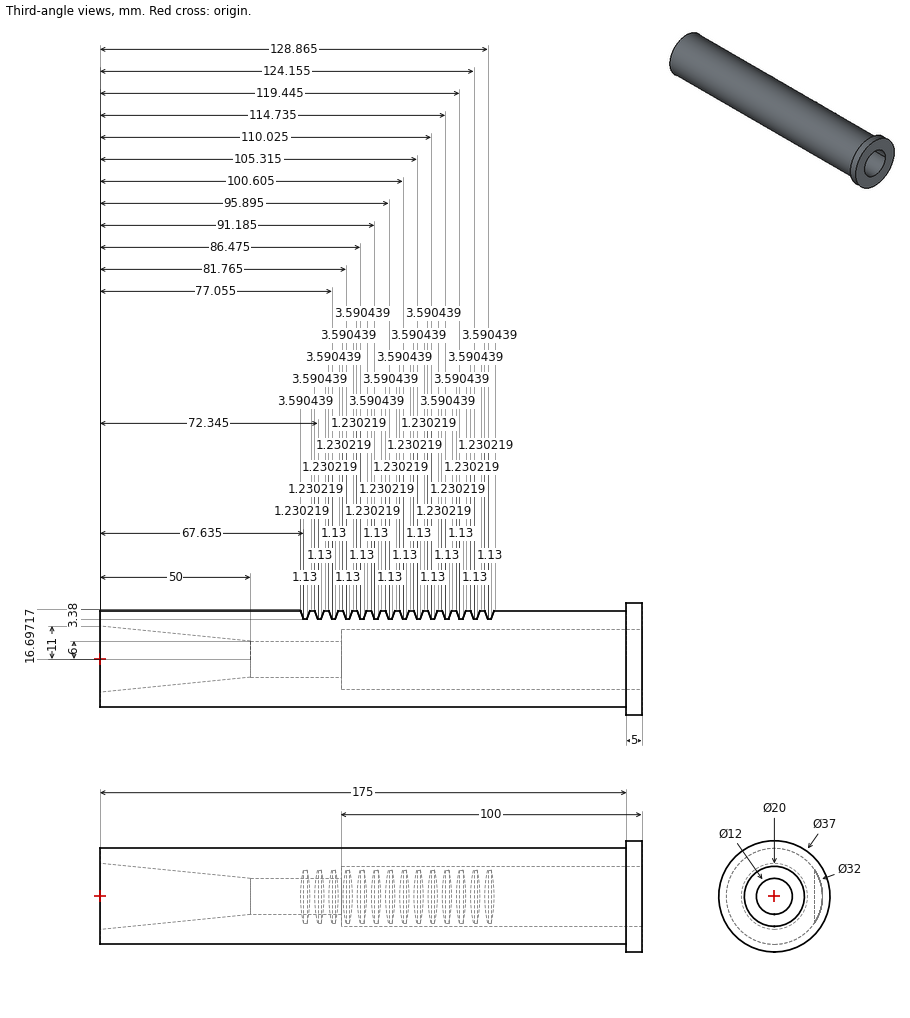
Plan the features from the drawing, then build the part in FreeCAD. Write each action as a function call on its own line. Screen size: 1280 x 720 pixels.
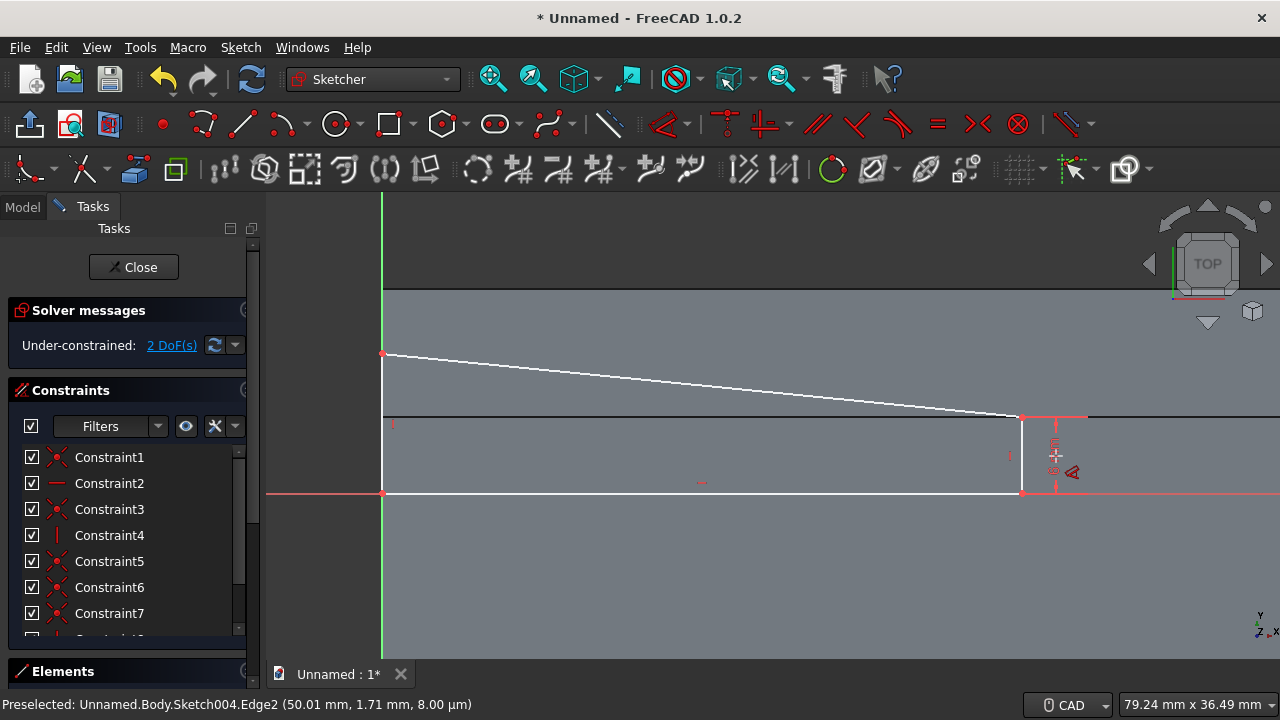
click(574, 494)
click(702, 528)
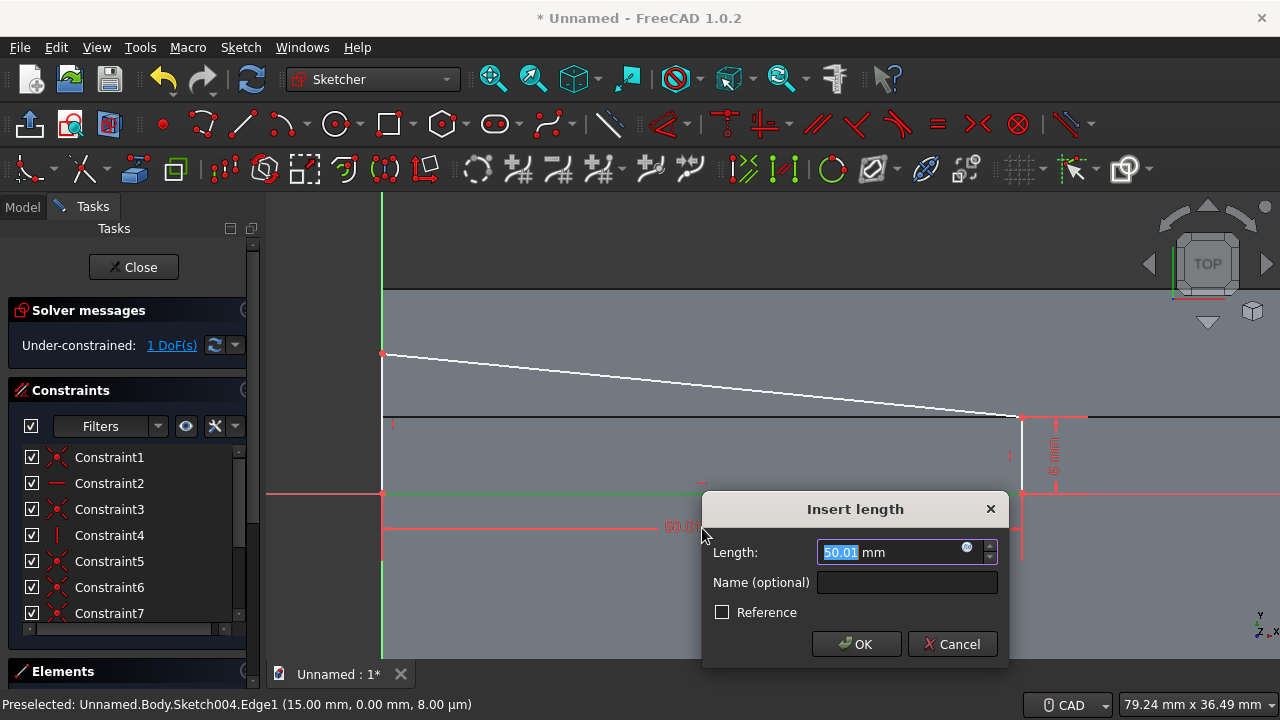
text(50)
key(Return)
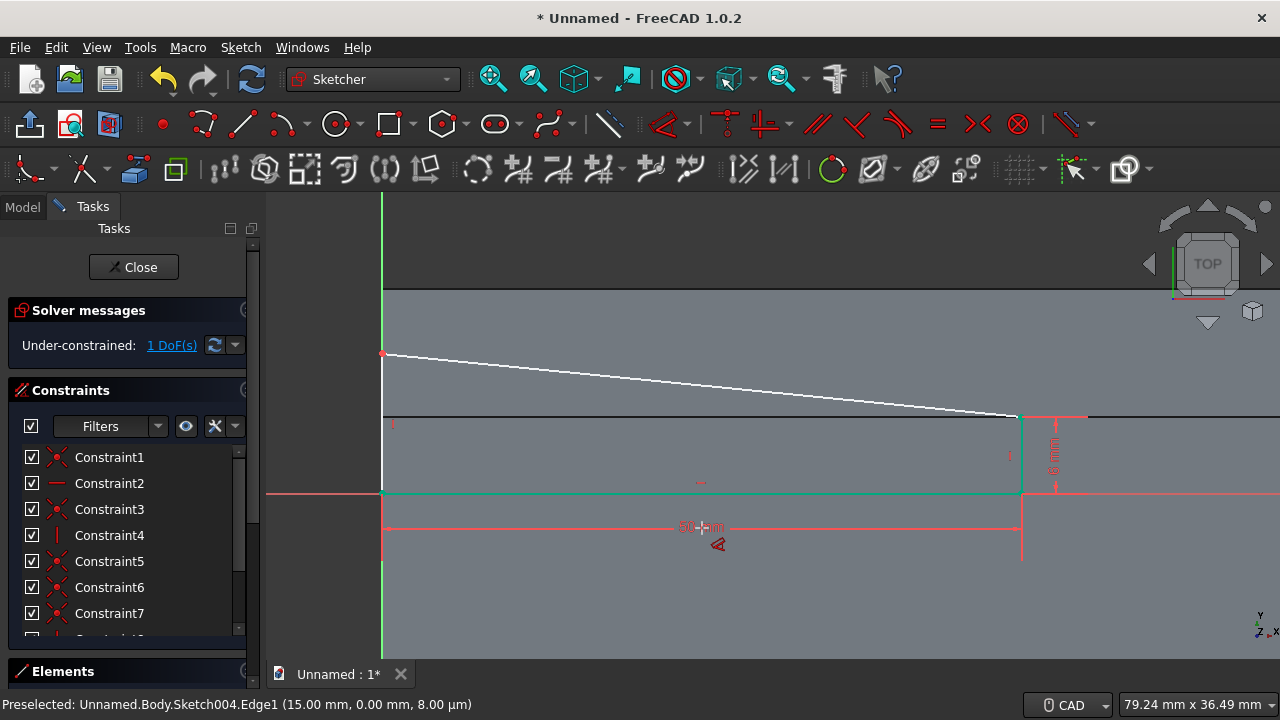
click(382, 396)
click(348, 424)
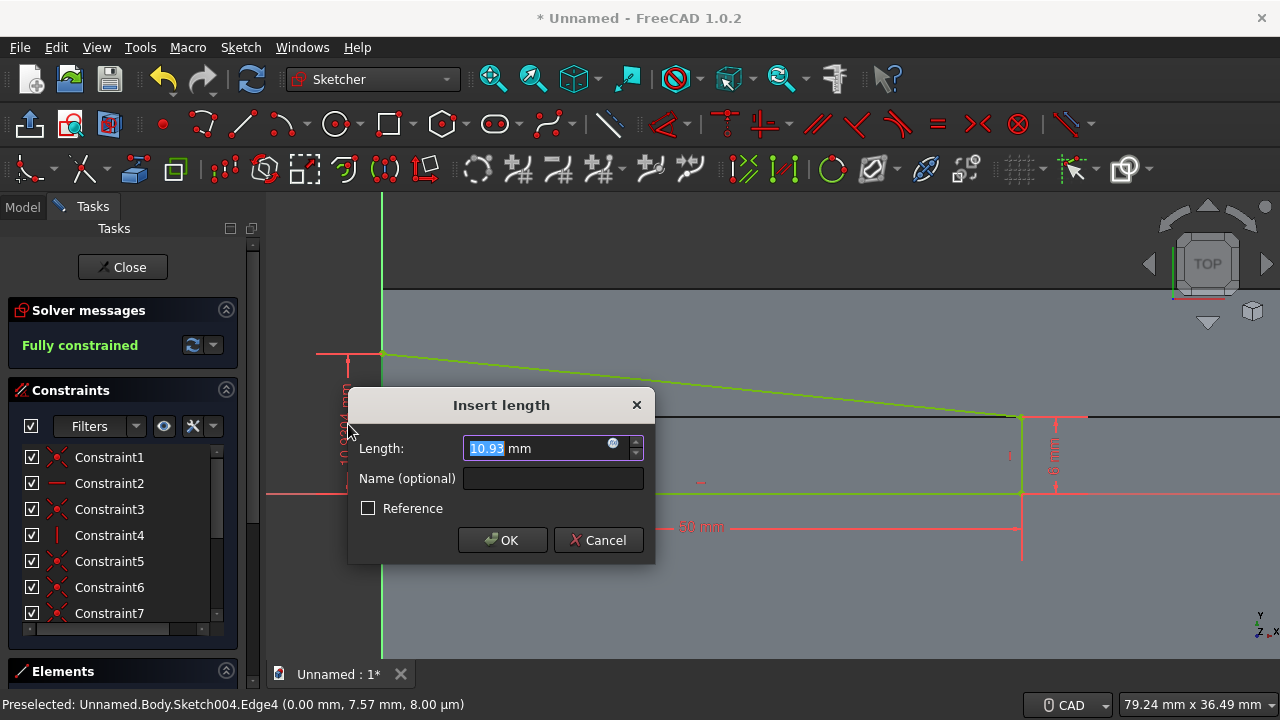
text(11)
key(Return)
key(Escape)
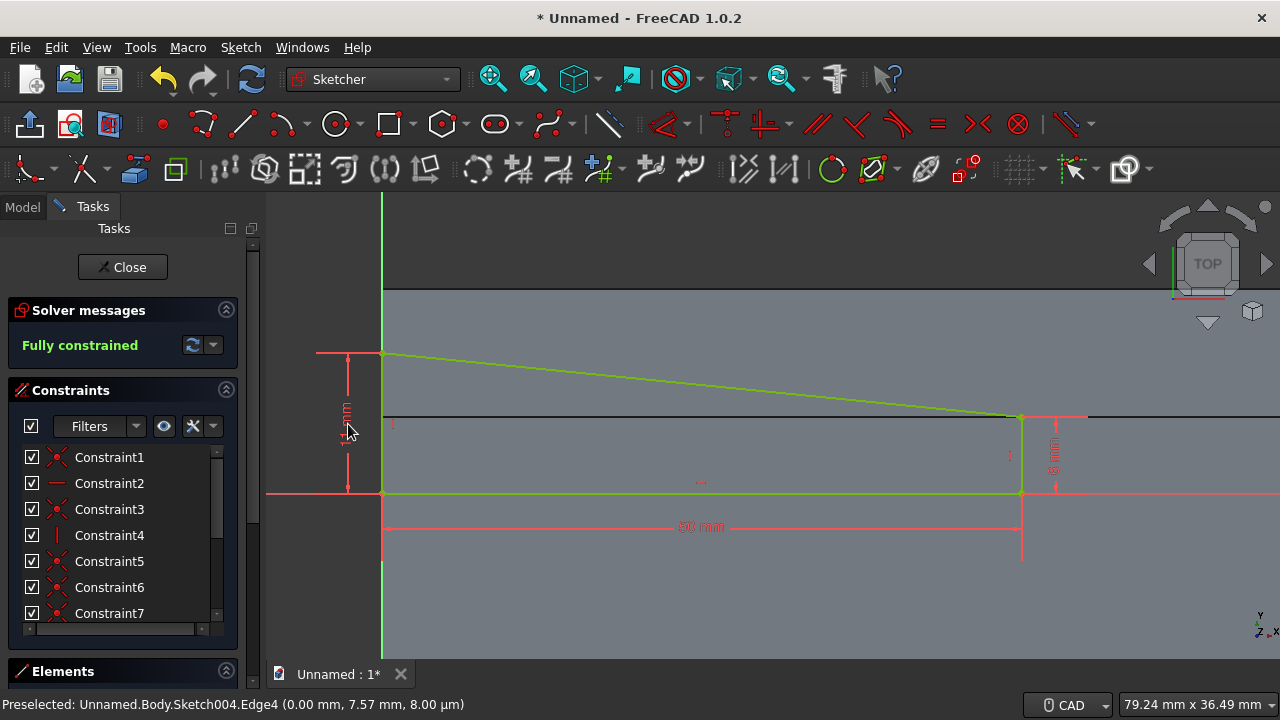
click(123, 267)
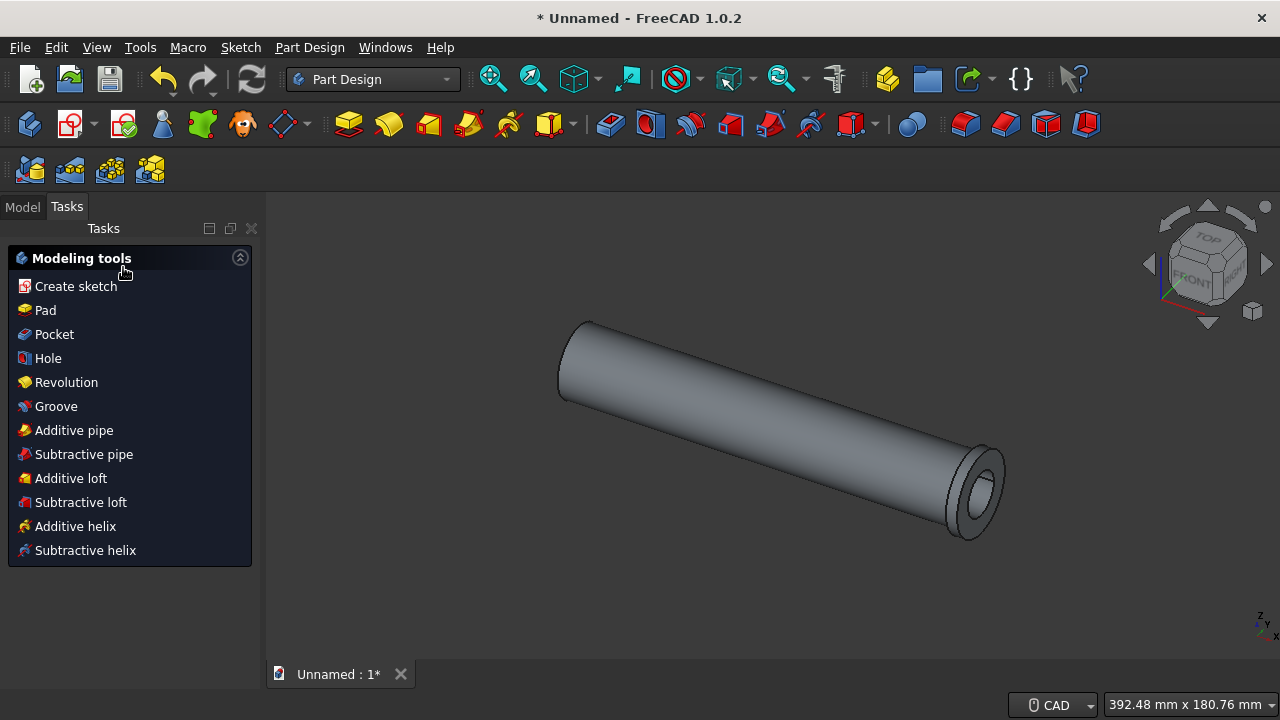
click(692, 124)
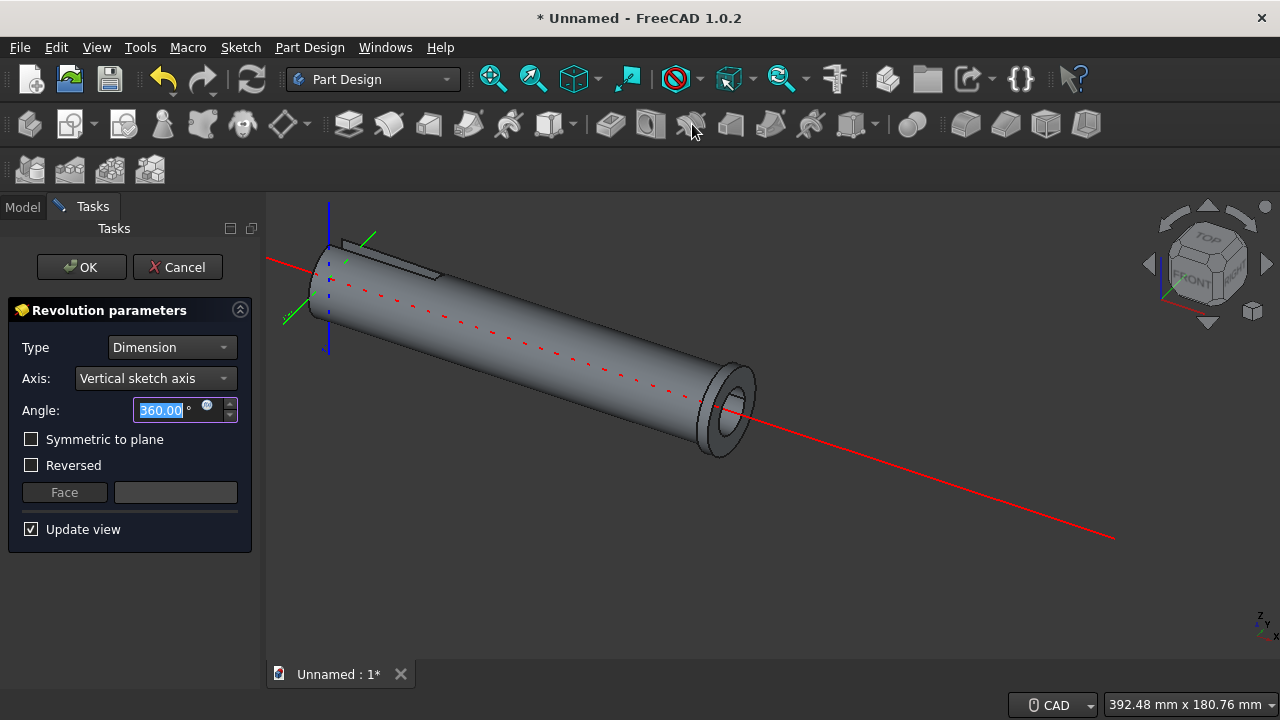
click(156, 378)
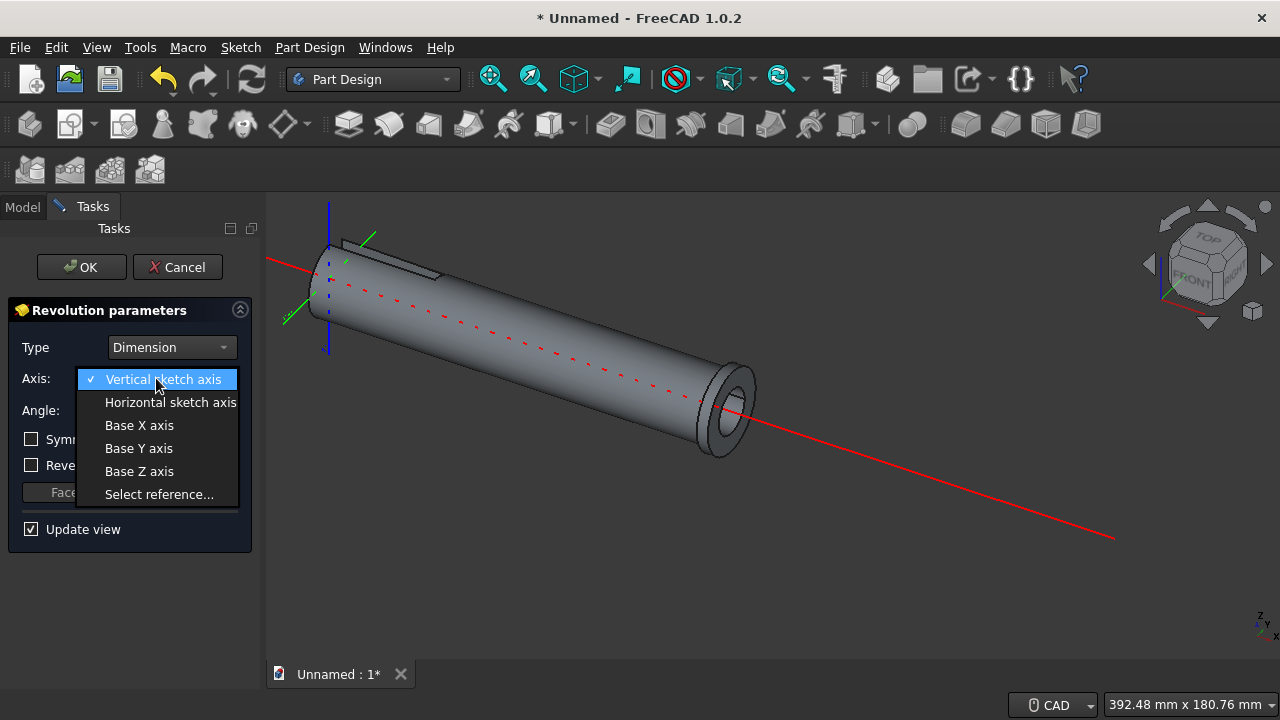
click(156, 402)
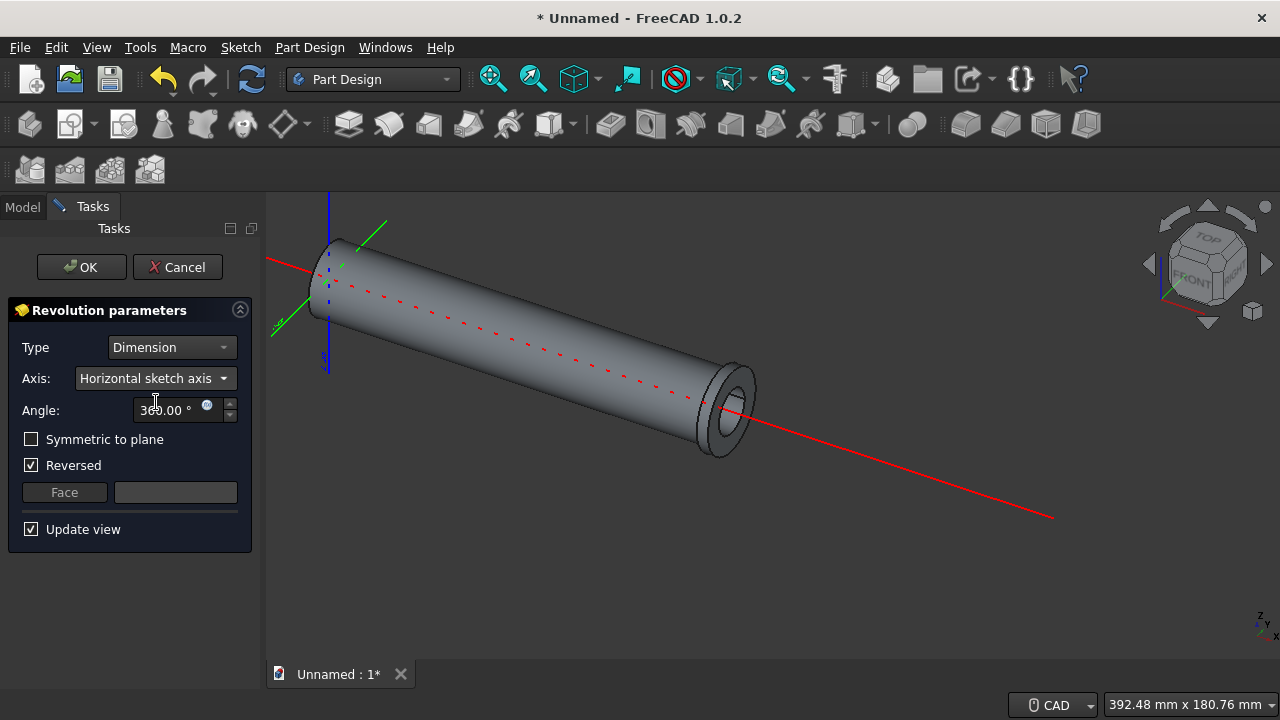
click(82, 267)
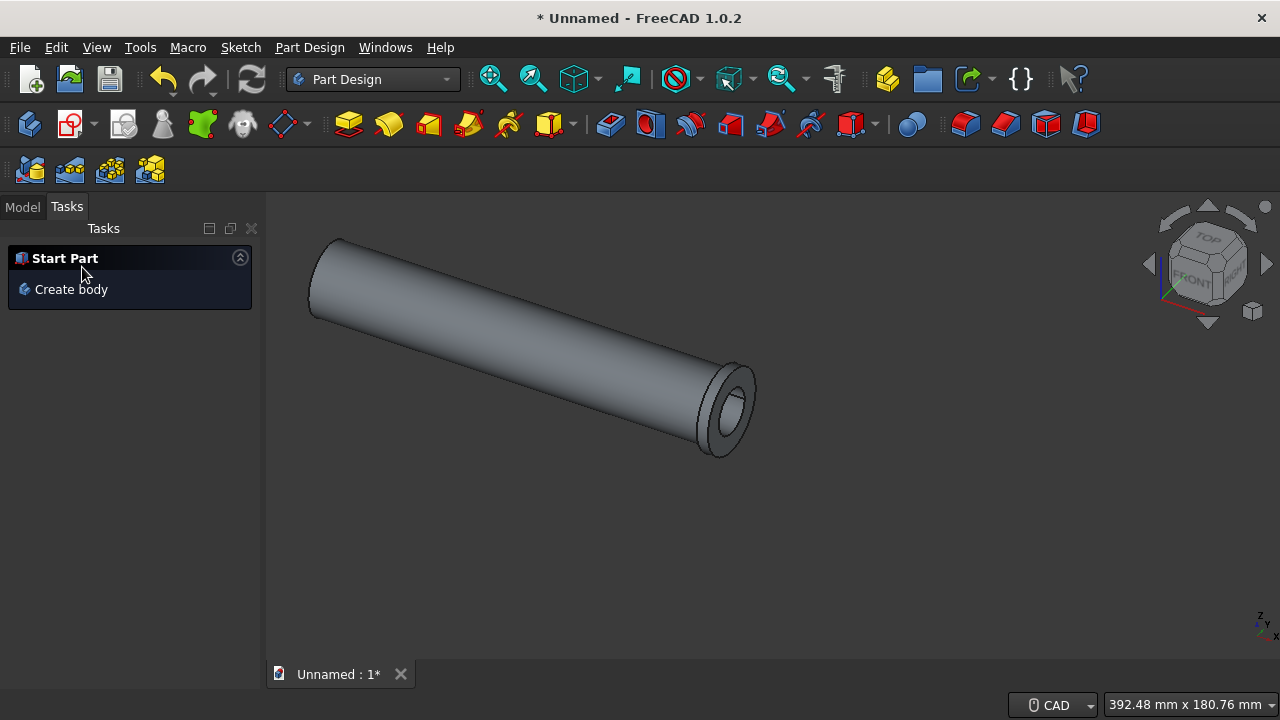
click(70, 124)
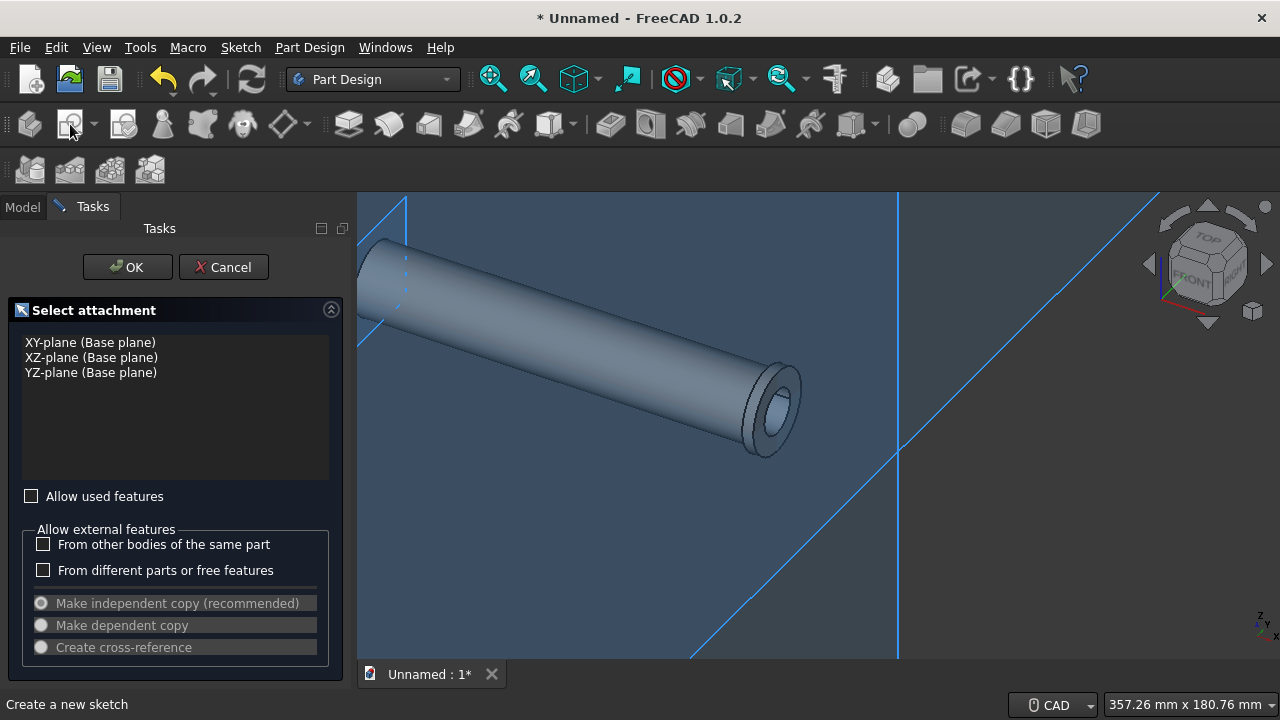
click(82, 342)